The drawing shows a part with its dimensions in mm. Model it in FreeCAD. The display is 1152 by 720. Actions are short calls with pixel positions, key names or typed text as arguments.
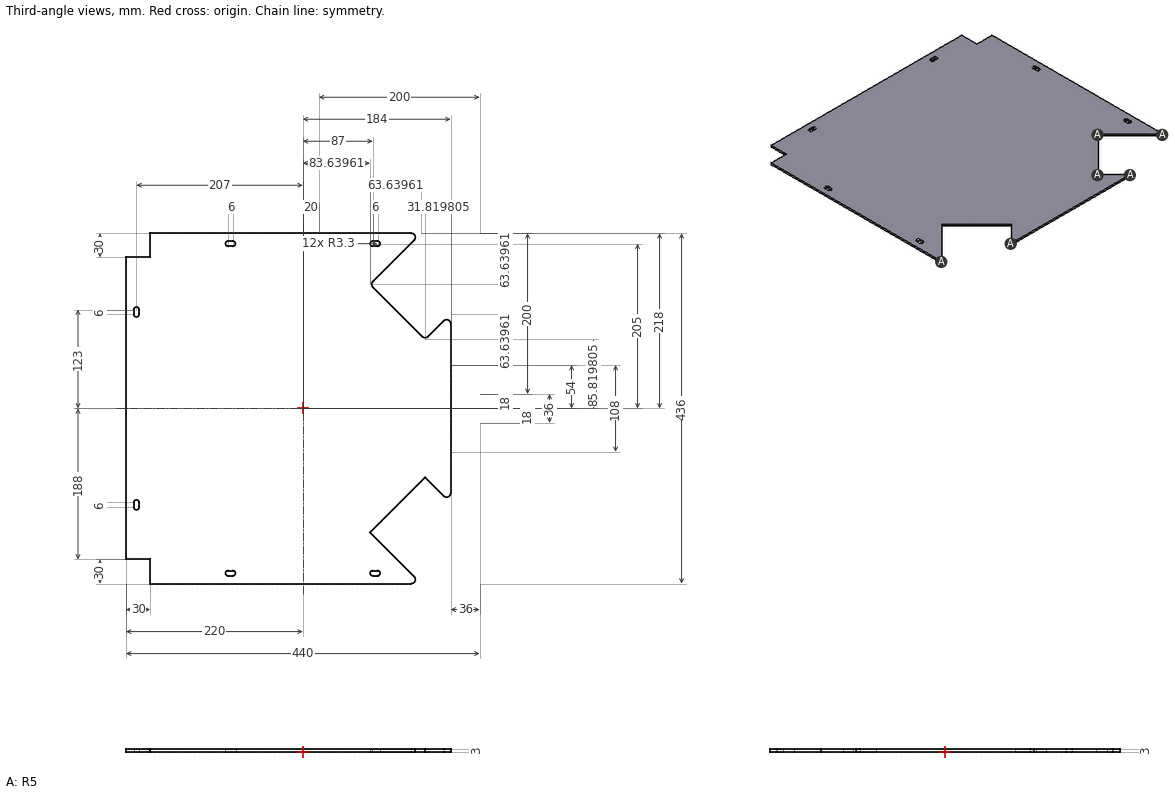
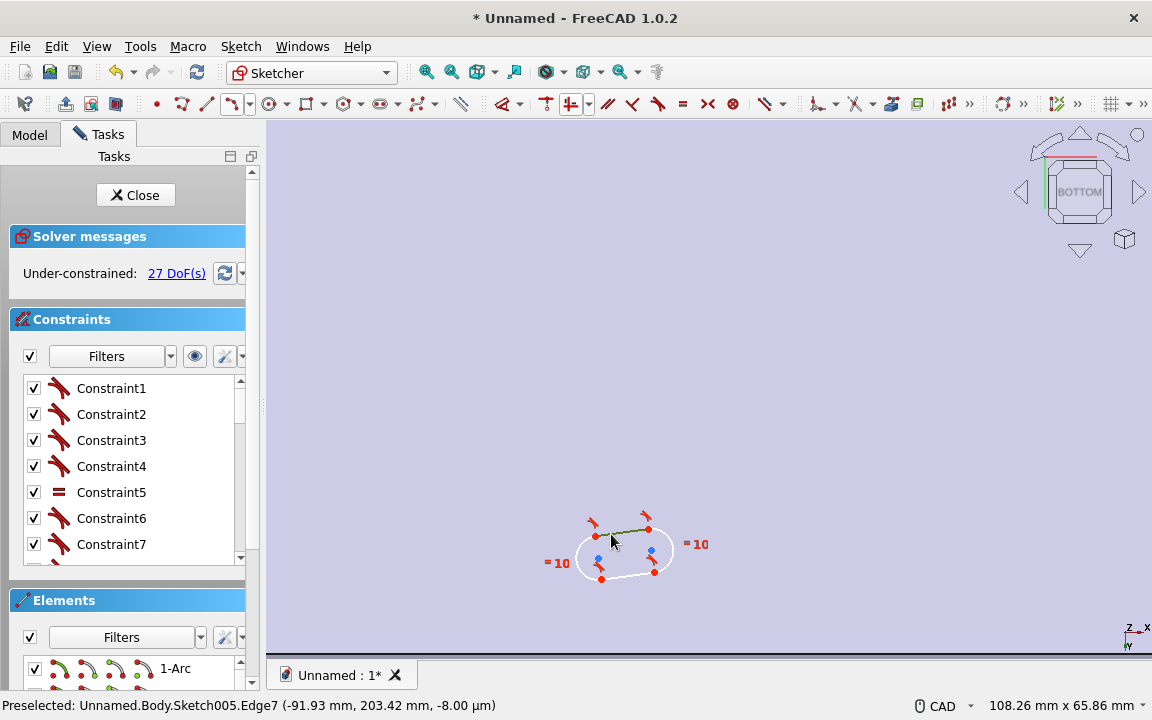
key(h)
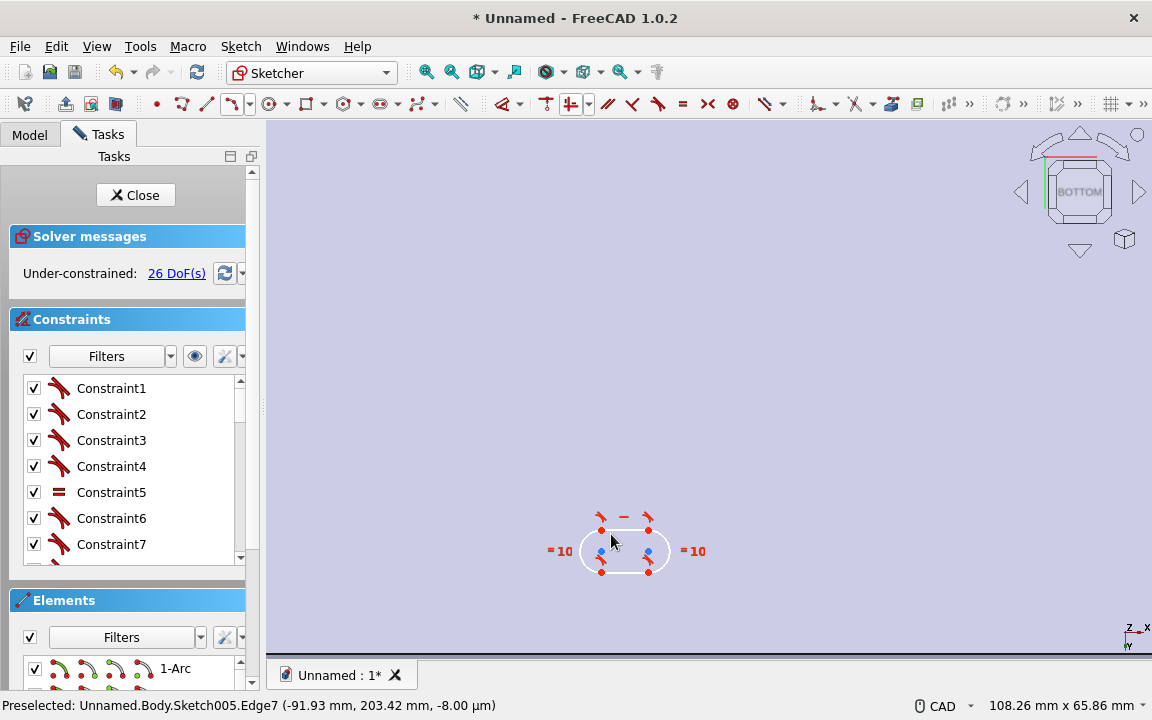
scroll(615, 541, down, 12)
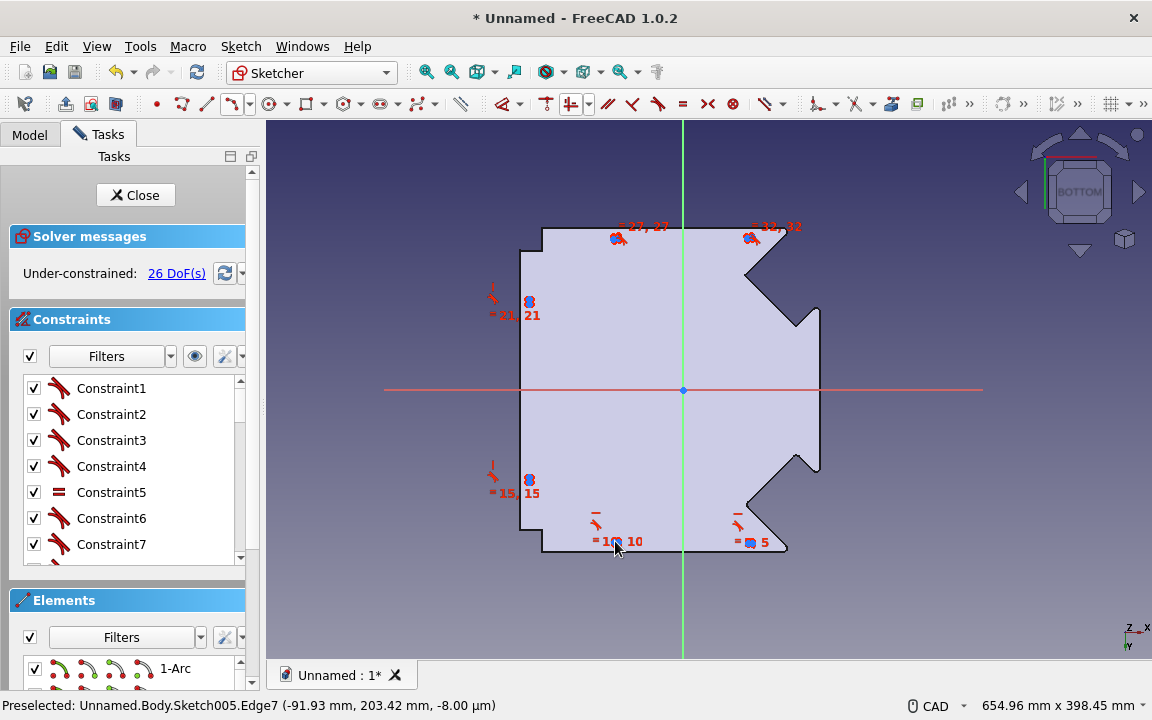
scroll(615, 236, up, 12)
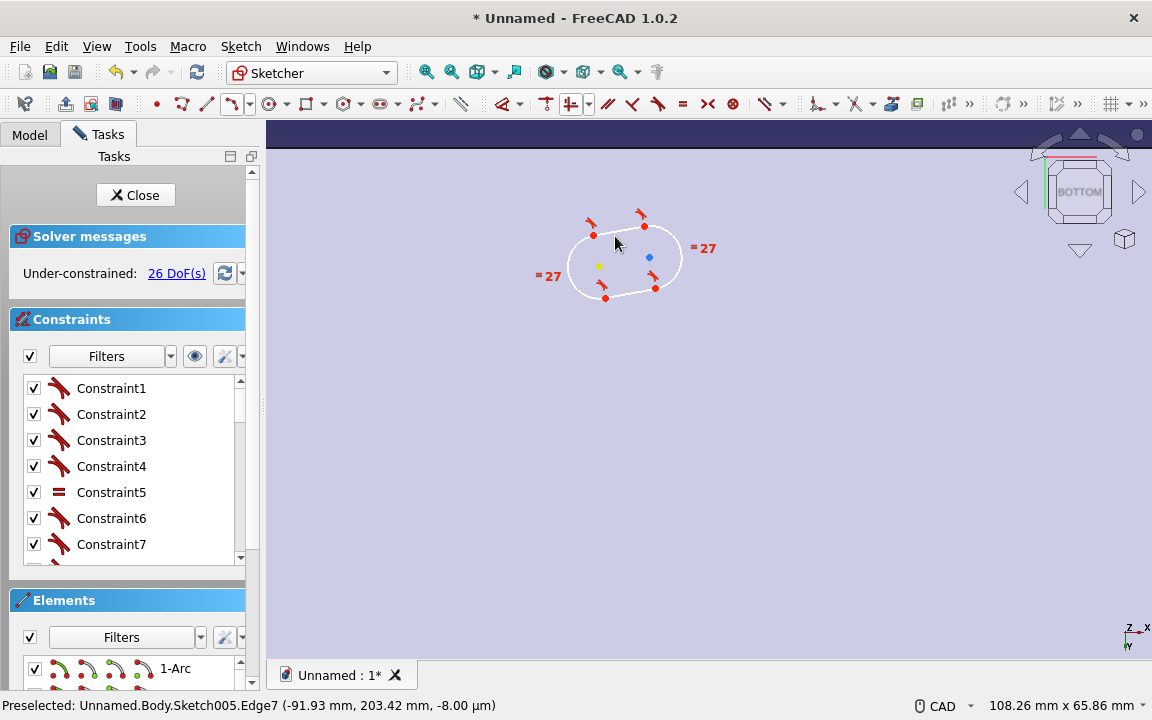
click(609, 233)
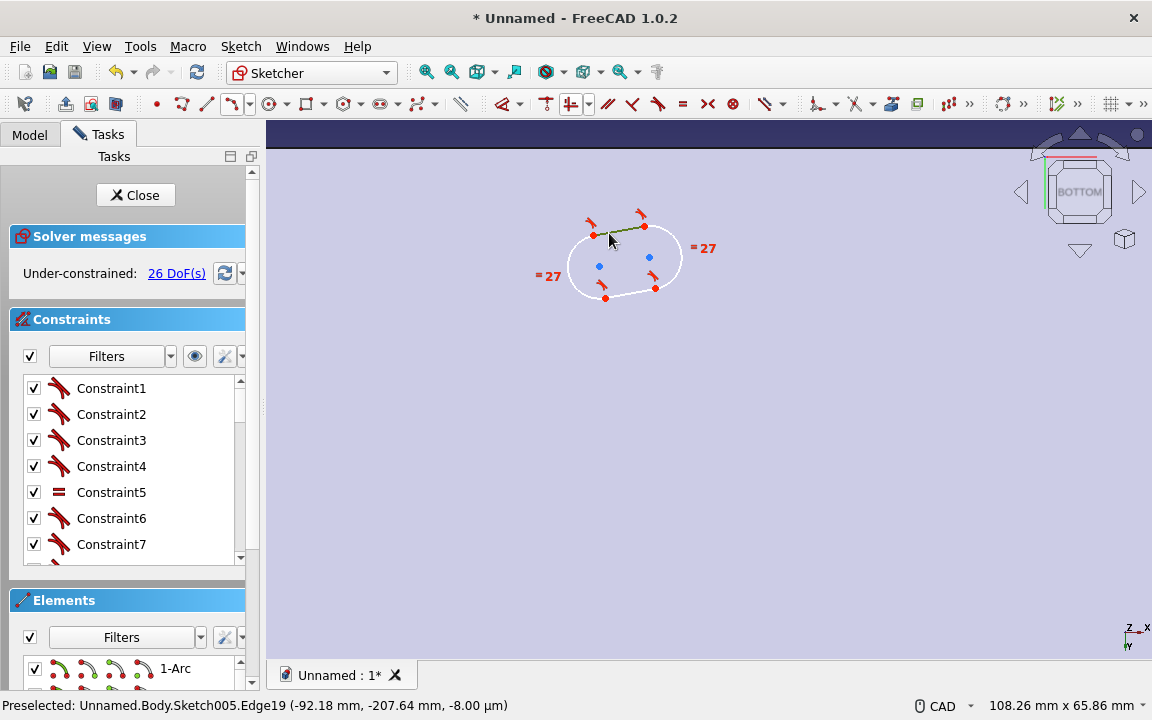
key(h)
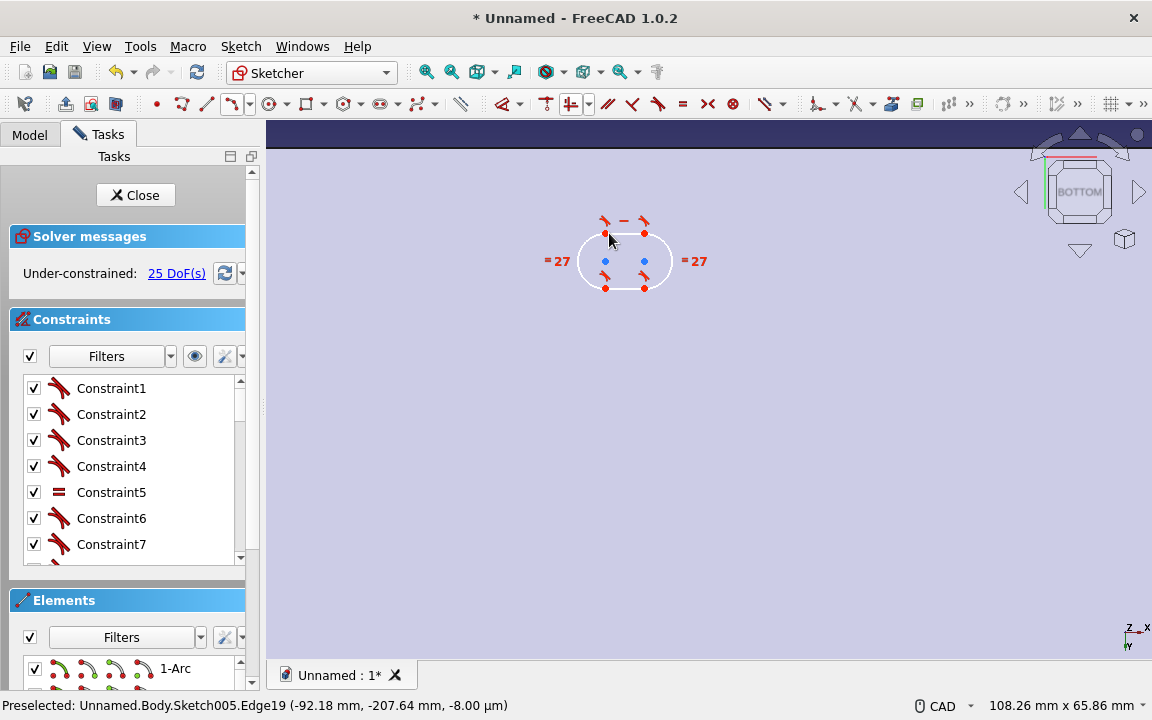
scroll(615, 236, down, 12)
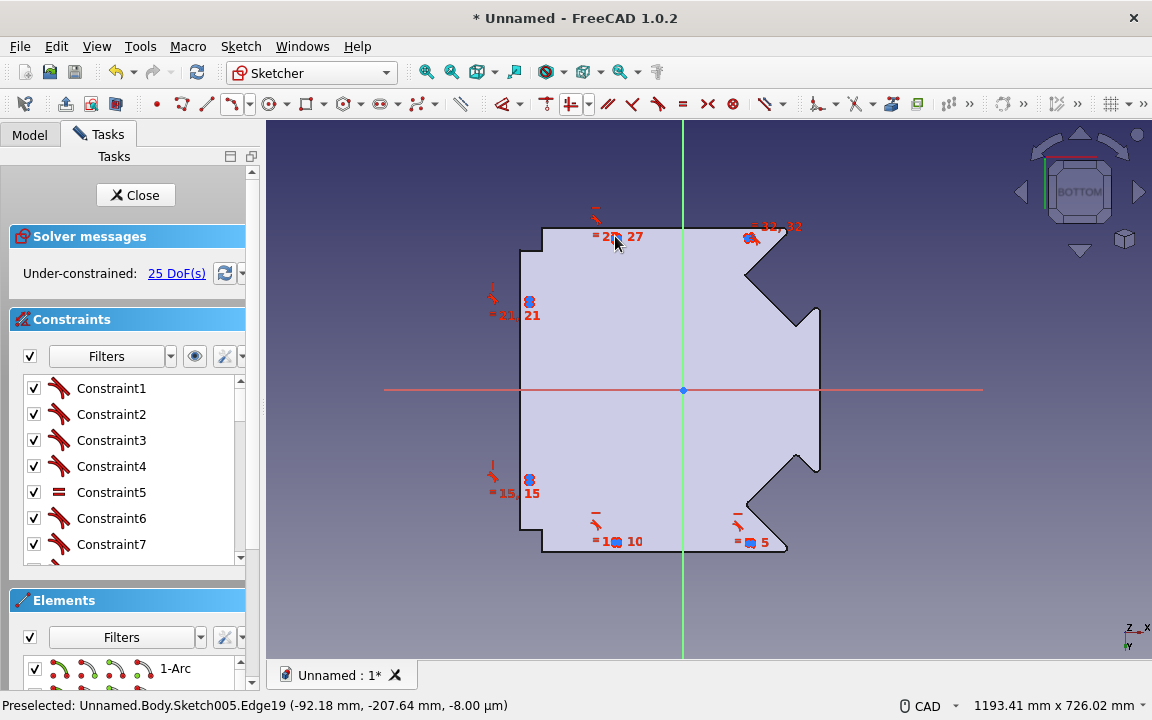
scroll(748, 236, up, 12)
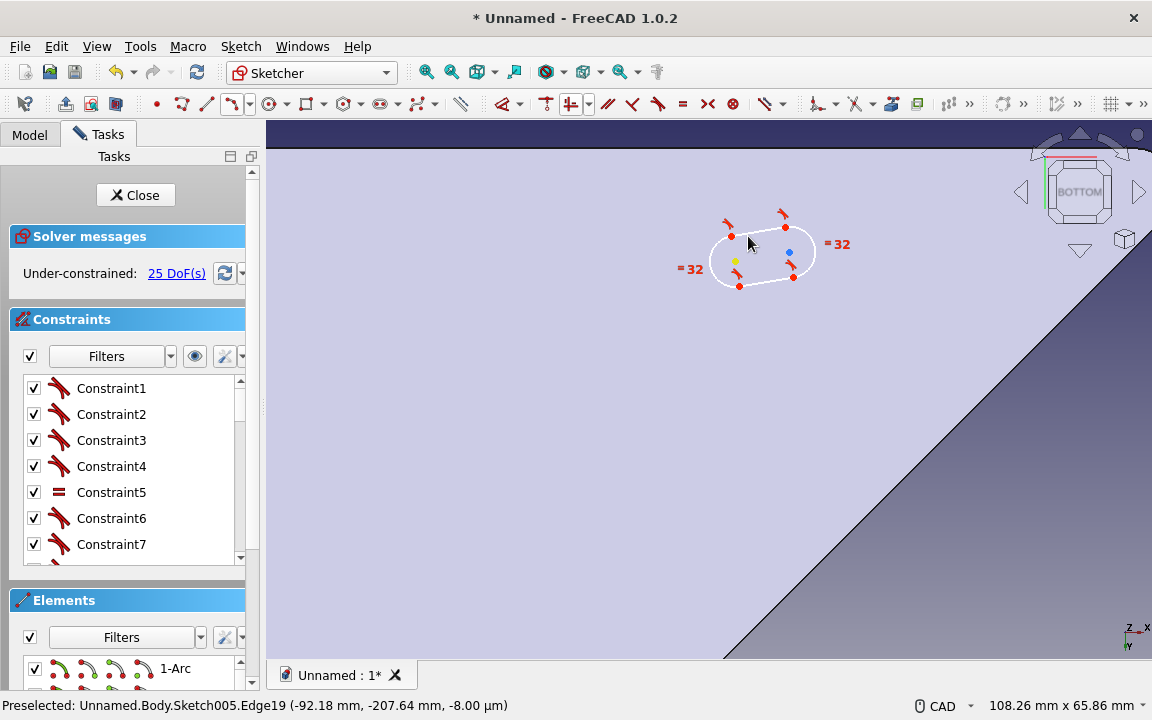
click(747, 234)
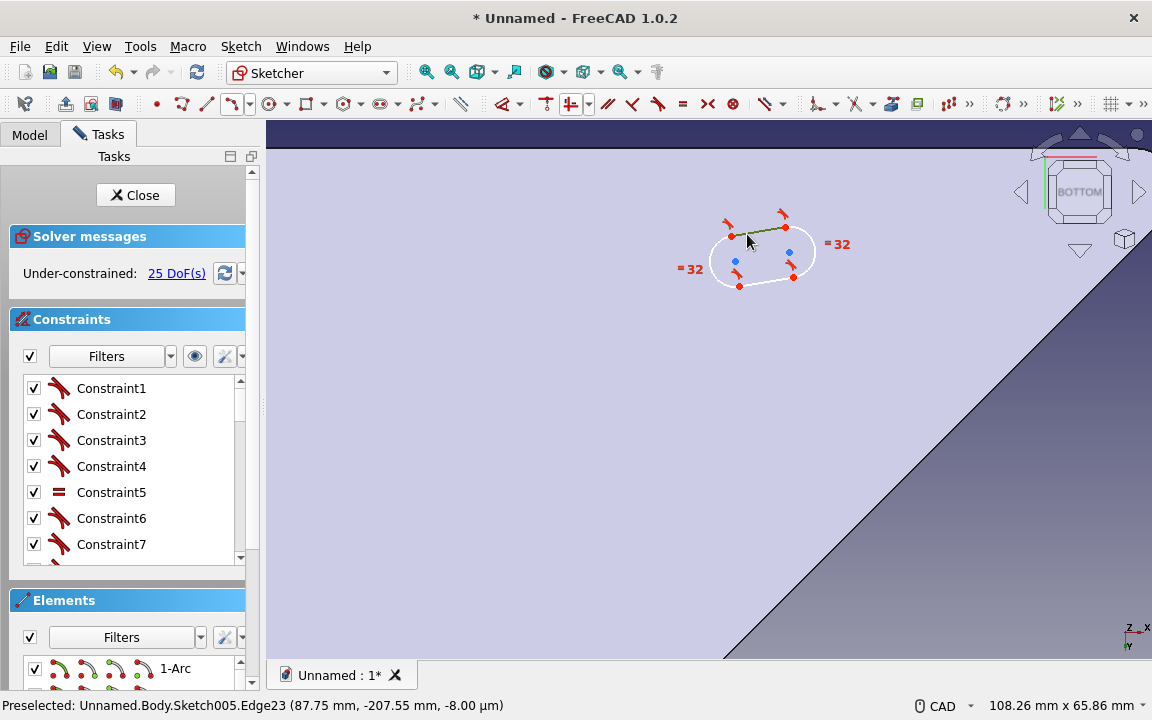
click(588, 104)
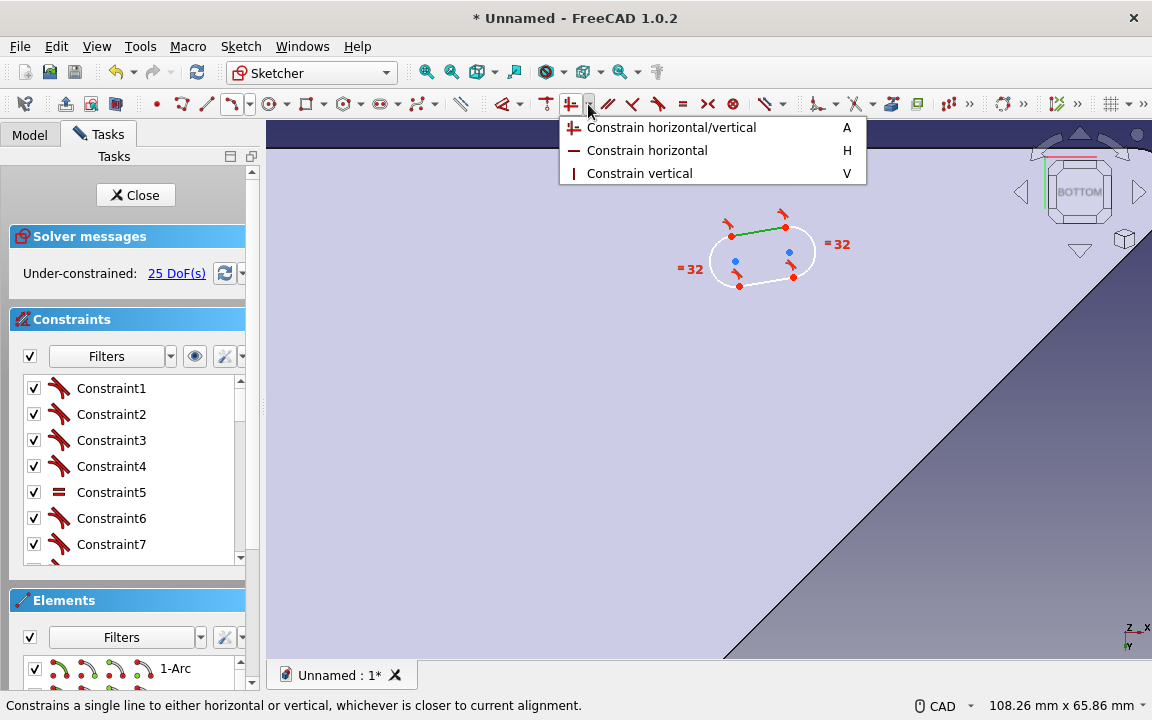
click(713, 150)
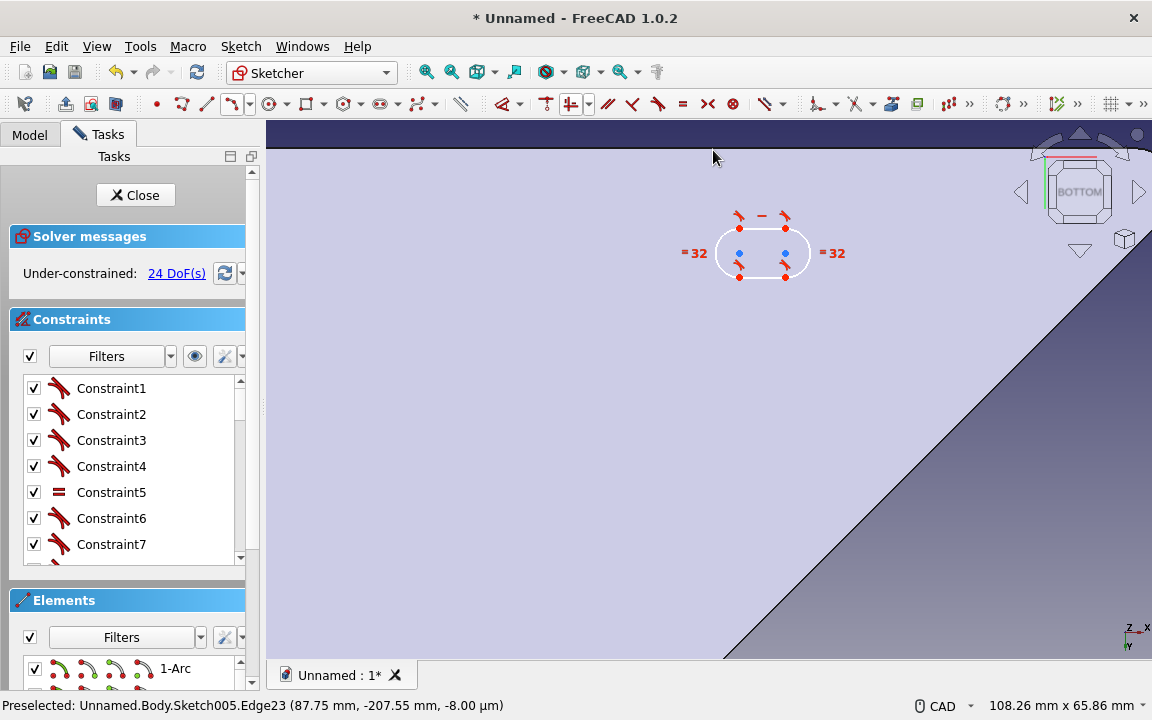
scroll(748, 236, down, 12)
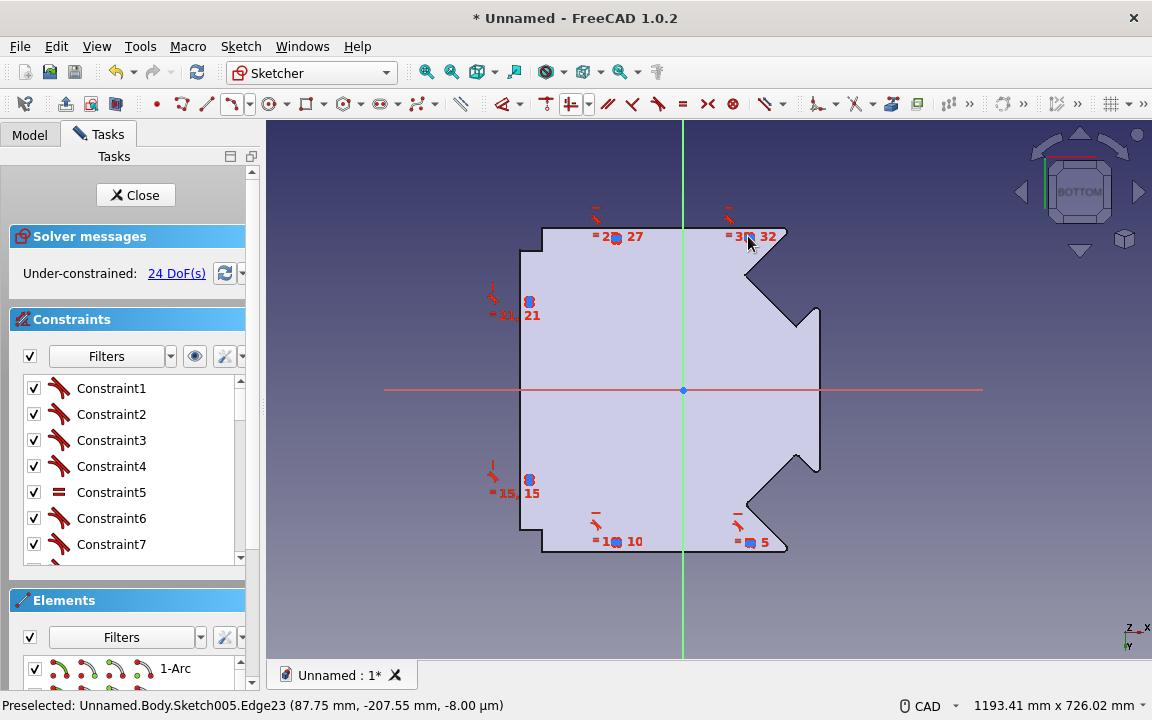
scroll(747, 542, up, 13)